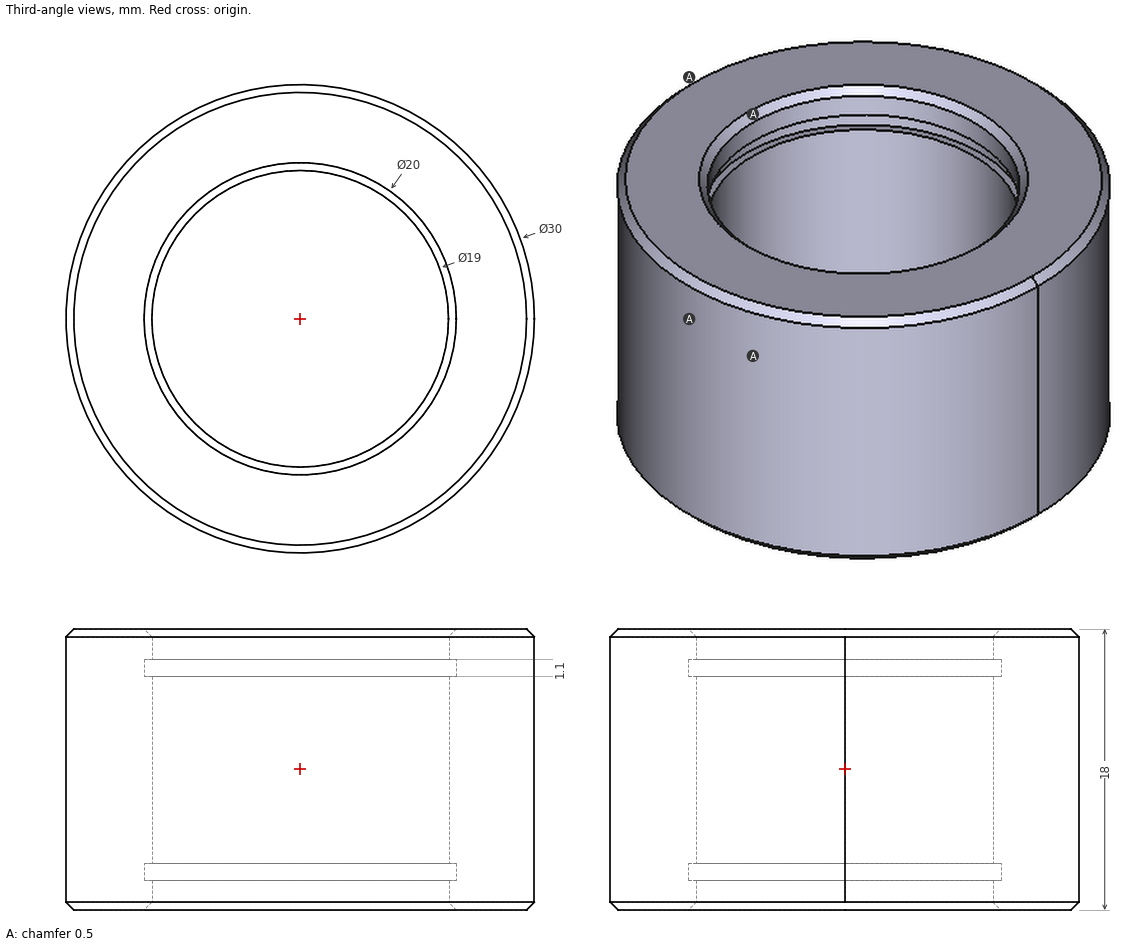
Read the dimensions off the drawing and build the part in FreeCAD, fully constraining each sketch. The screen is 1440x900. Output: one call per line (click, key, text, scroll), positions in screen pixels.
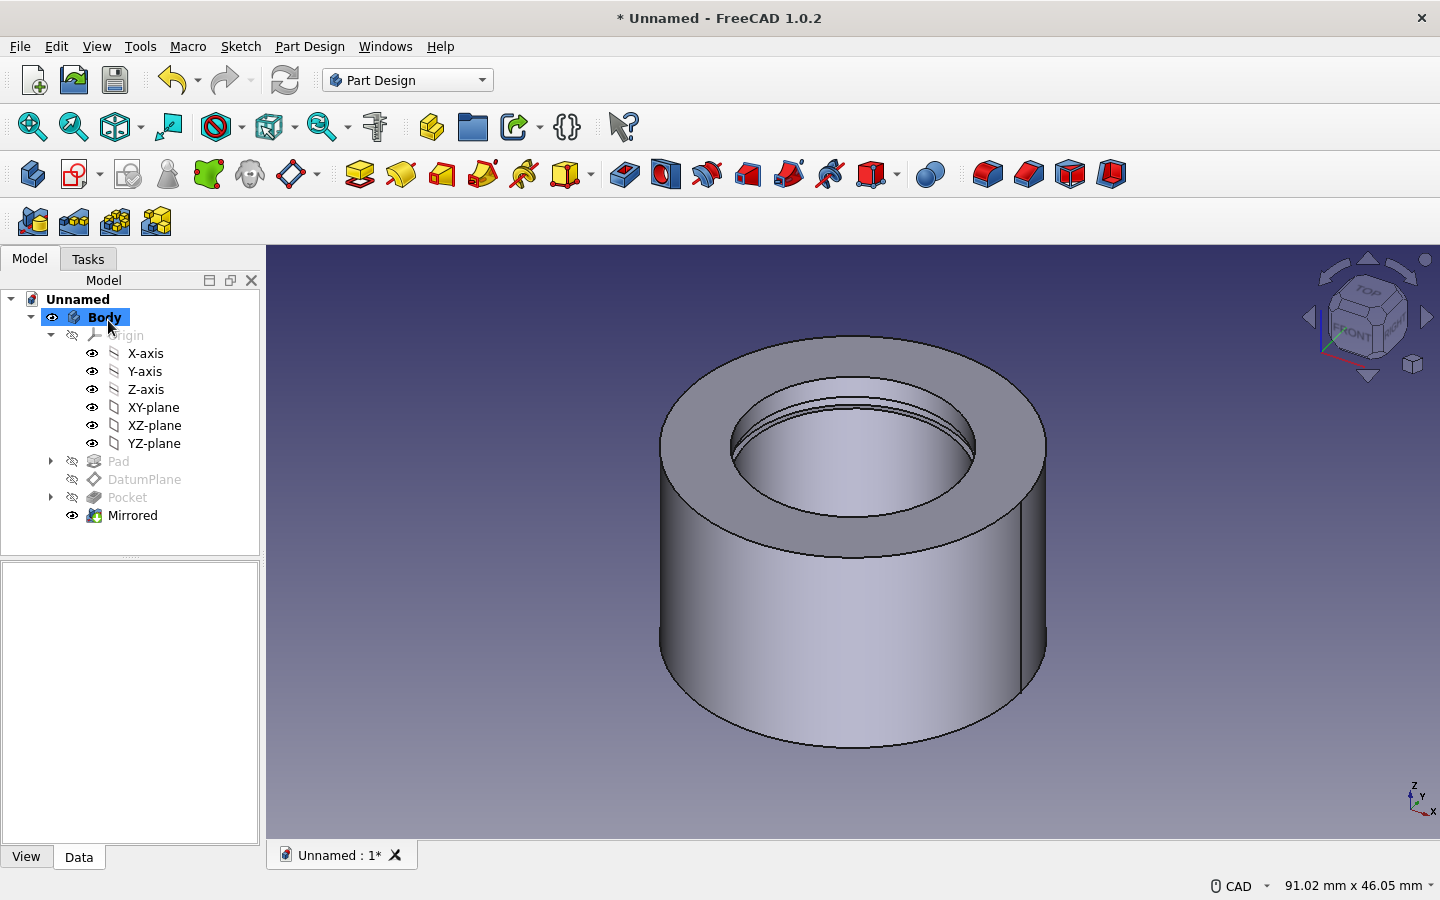
click(661, 458)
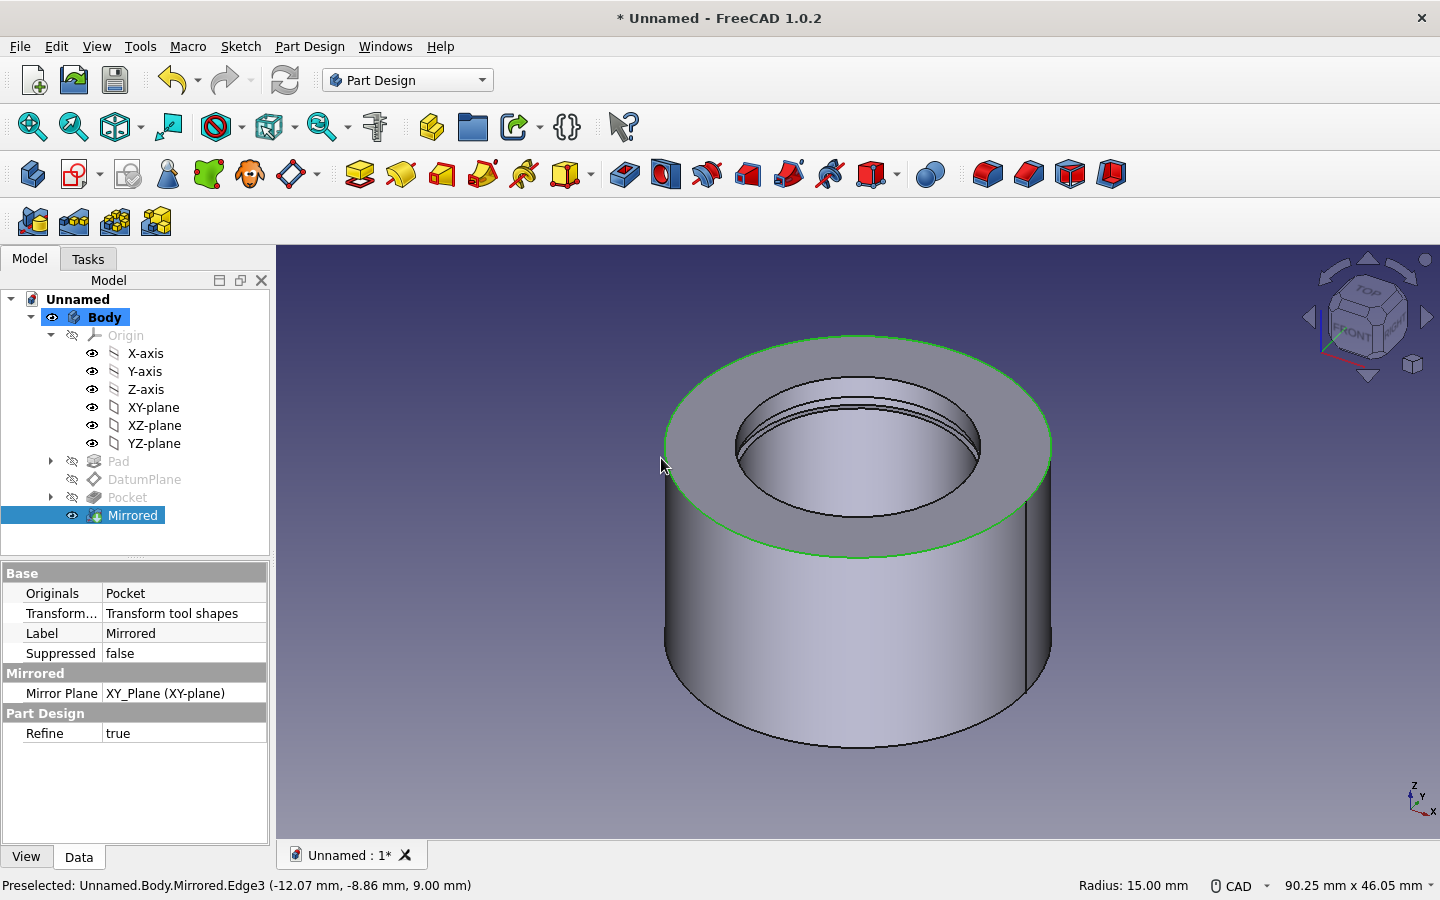
click(752, 411, ctrl)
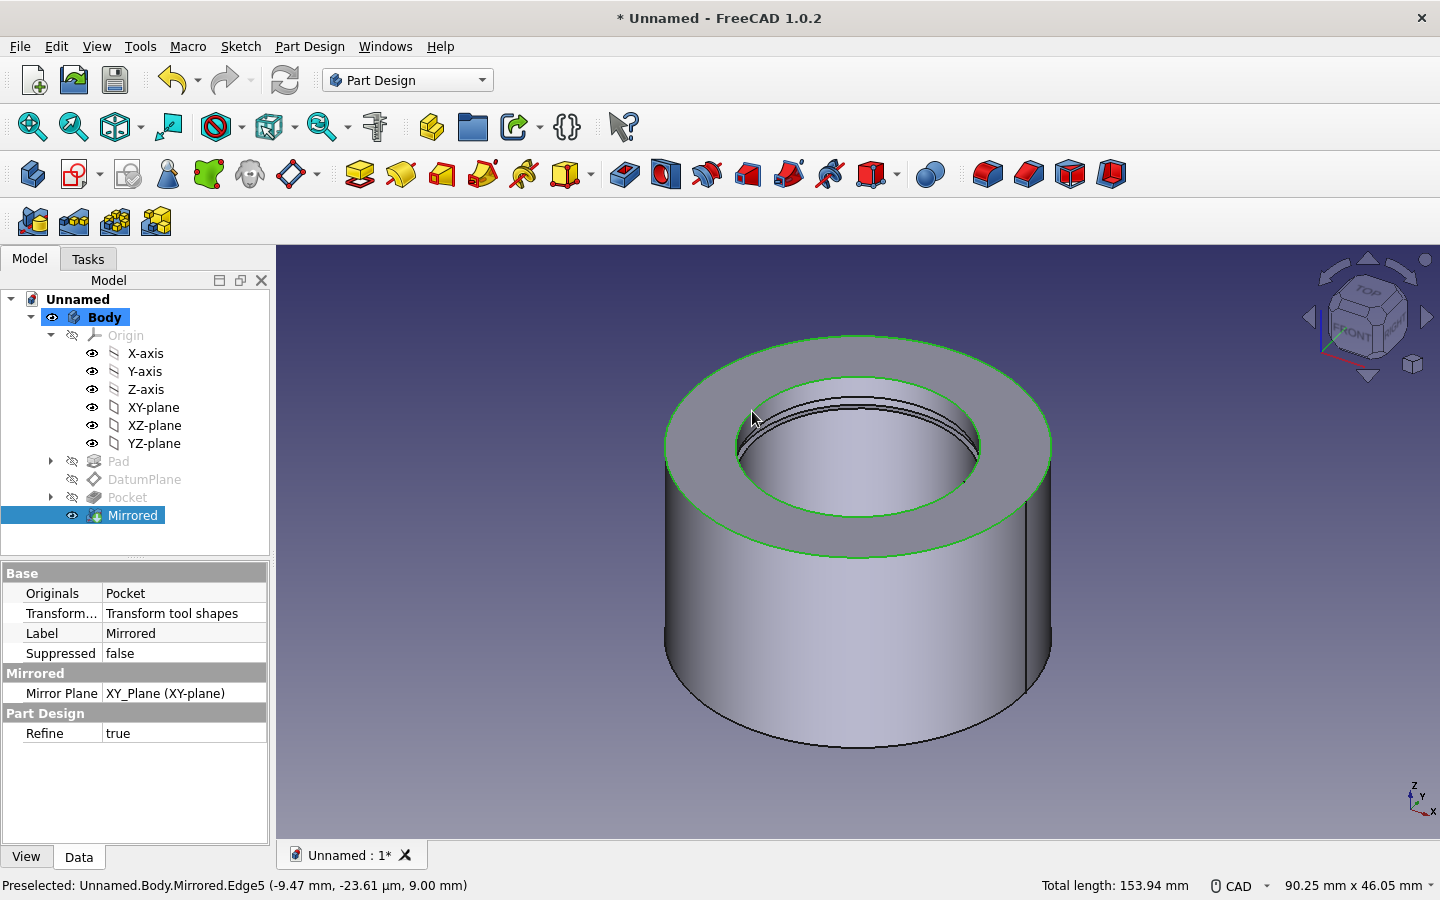
key(0)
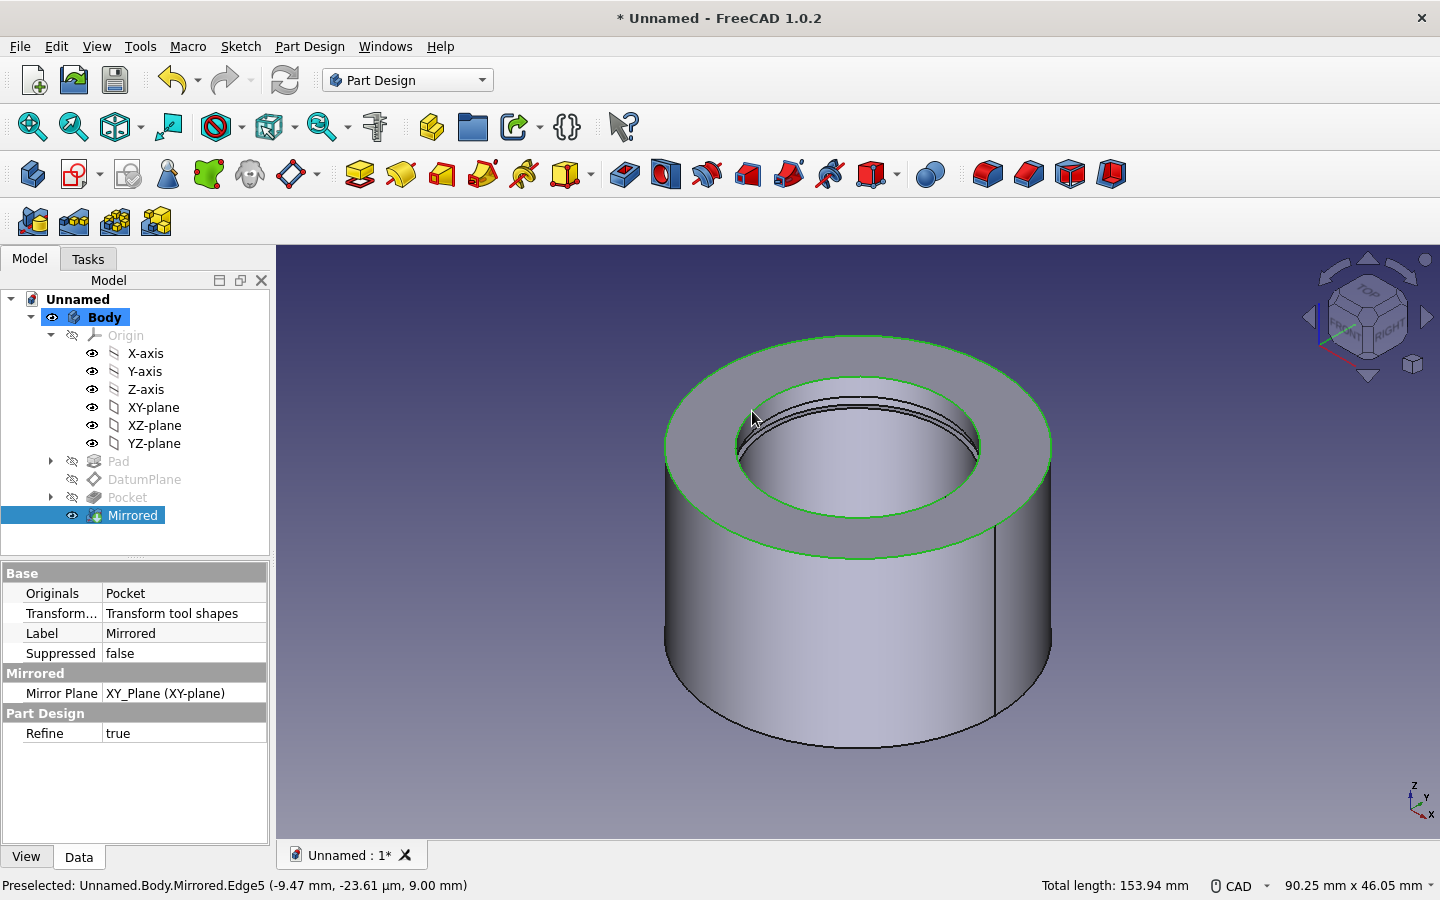
key(2)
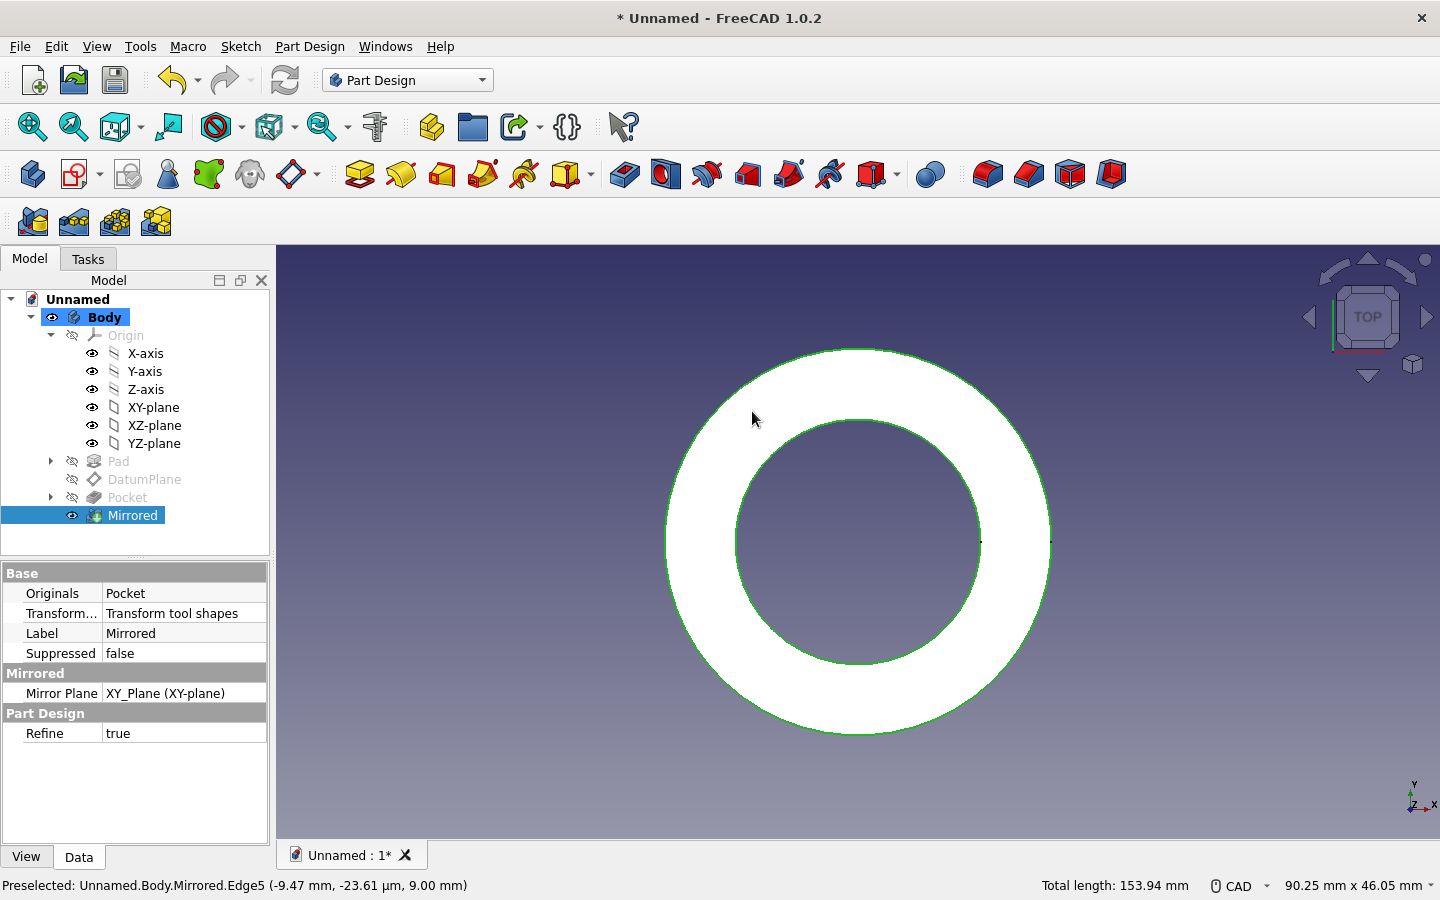
key(1)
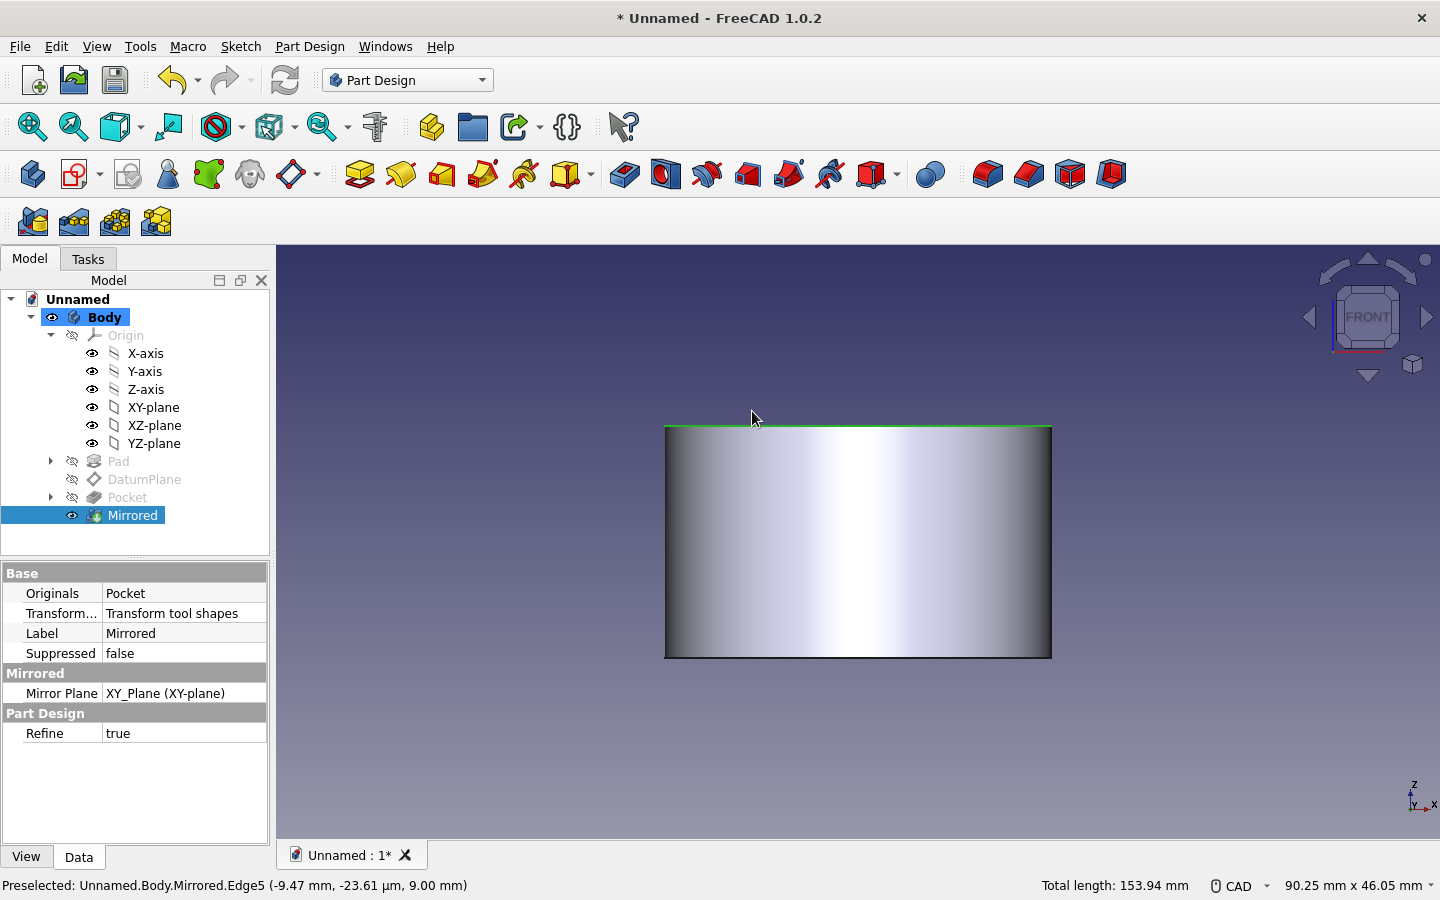
click(33, 128)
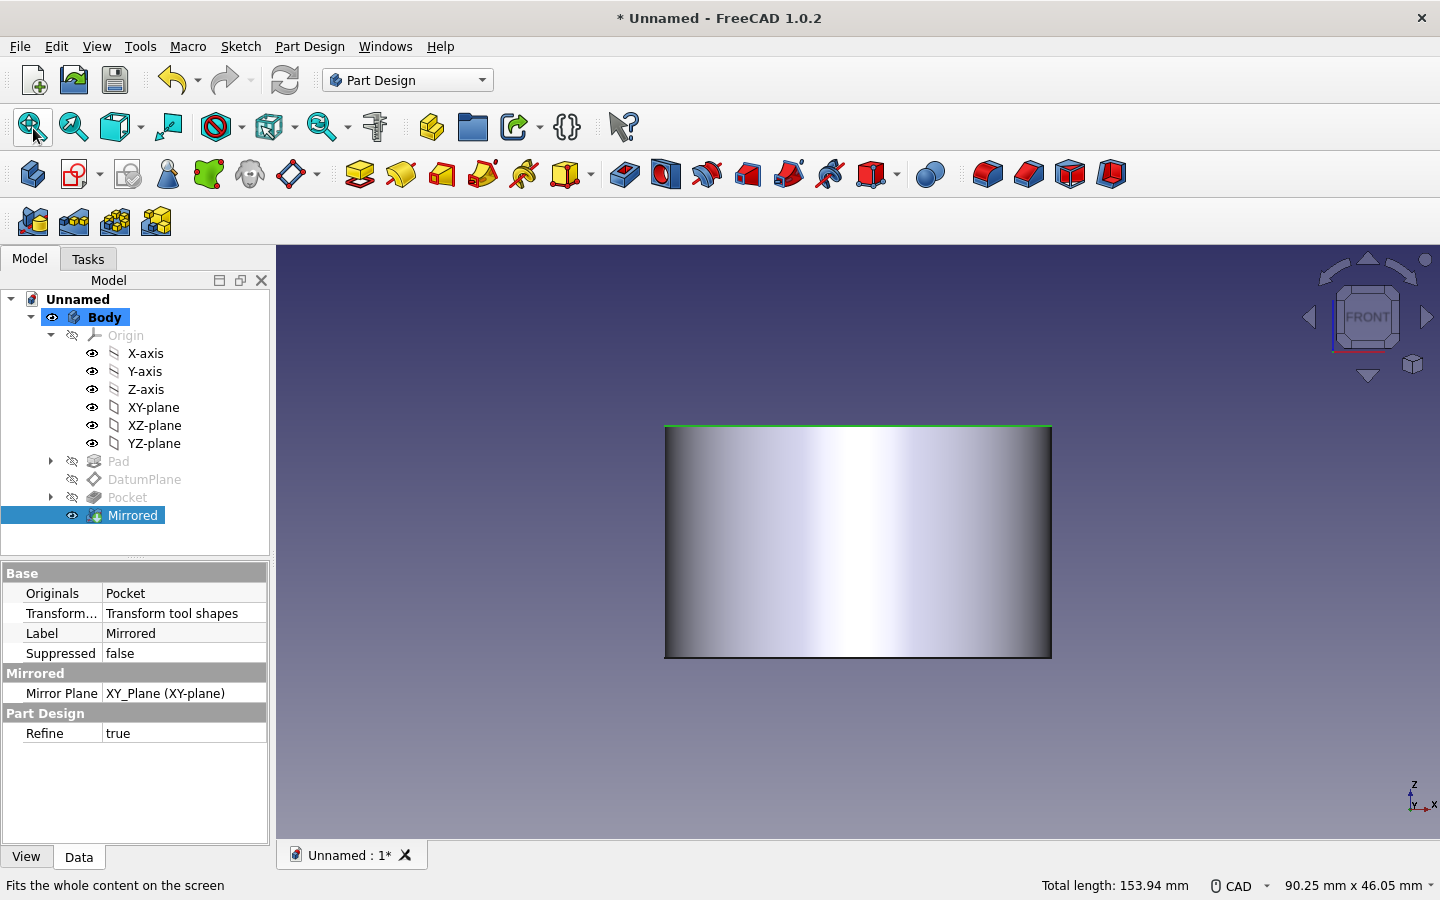
click(701, 657, ctrl)